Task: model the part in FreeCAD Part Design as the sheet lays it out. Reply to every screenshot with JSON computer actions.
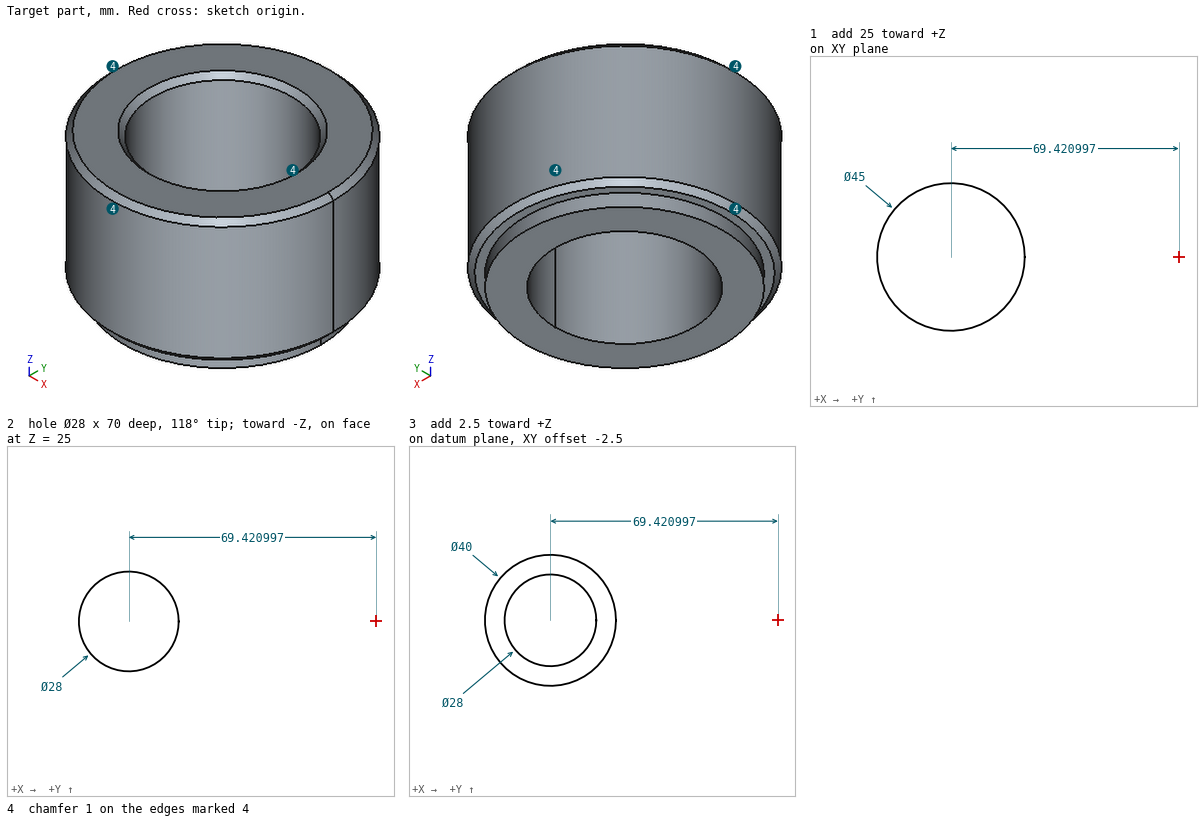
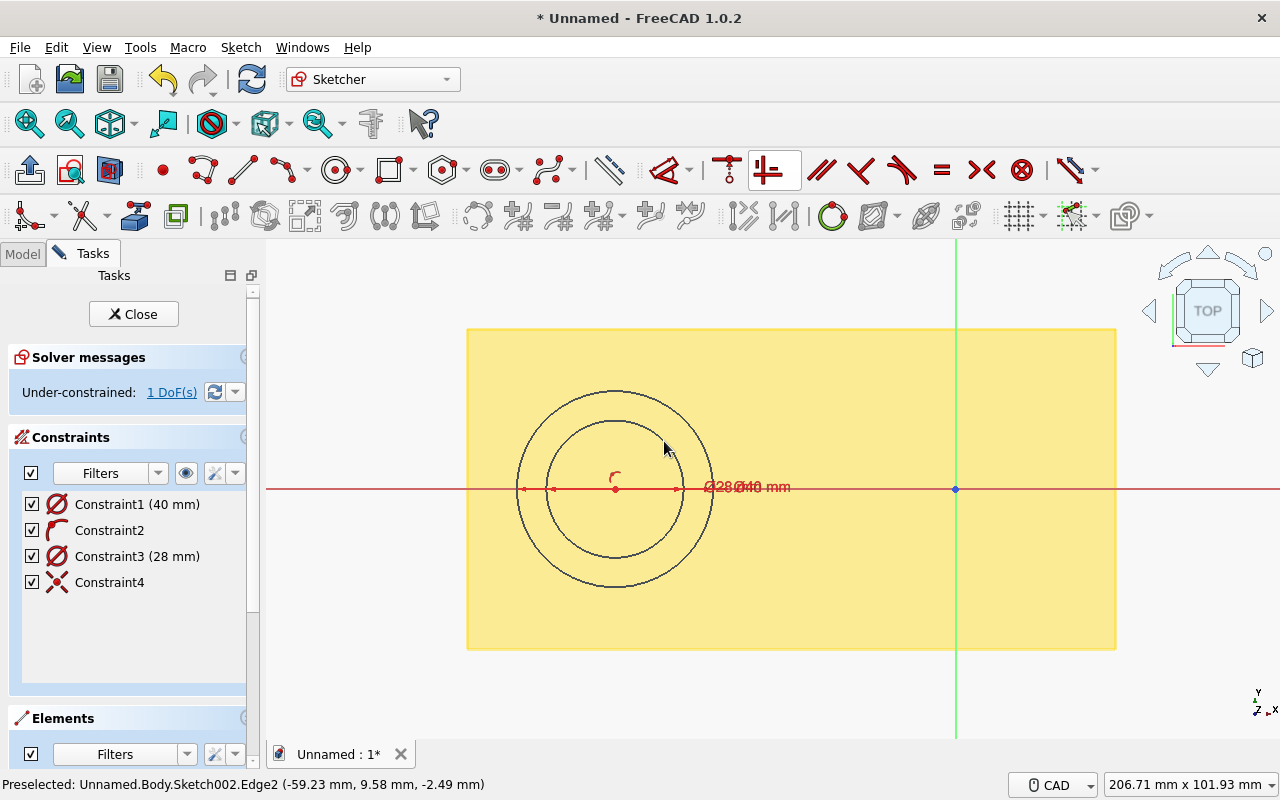
{"action": "key", "text": "d"}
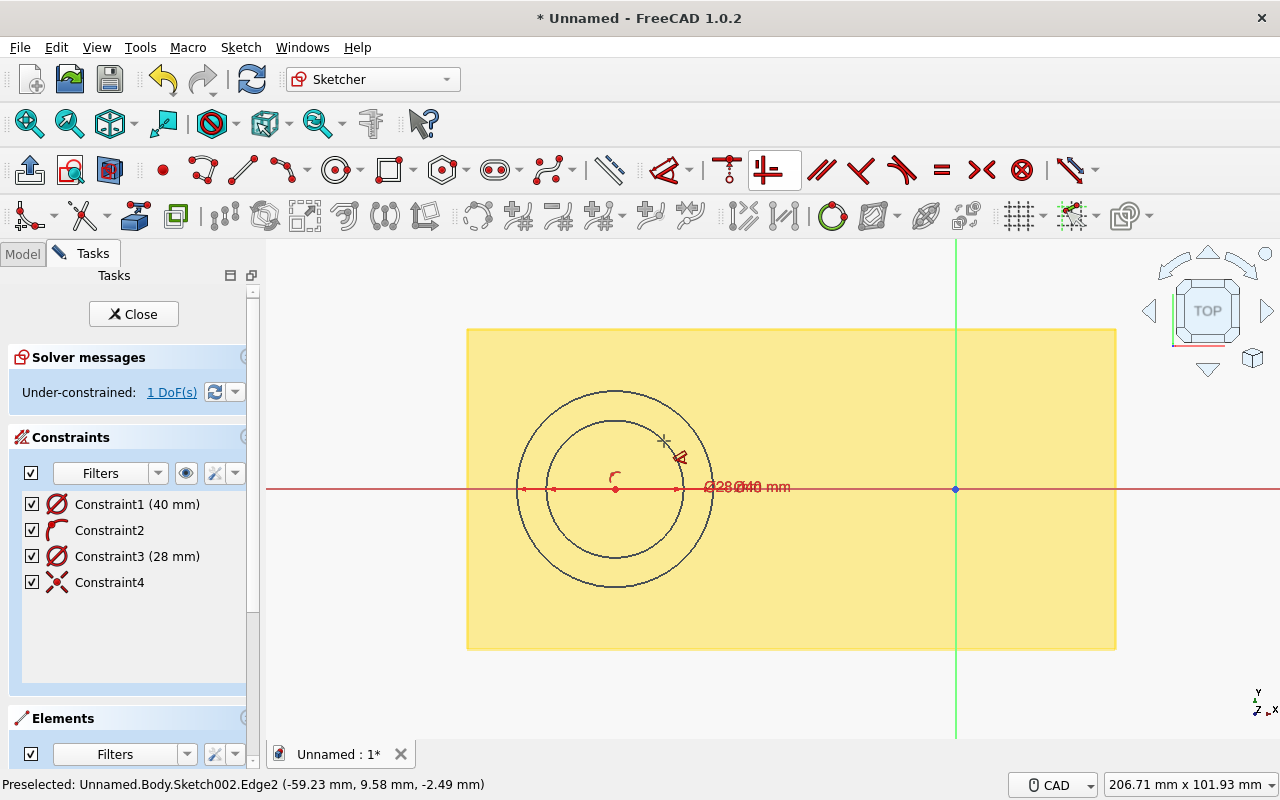
{"action": "left_click", "coordinate": [615, 489]}
{"action": "left_click", "coordinate": [785, 523]}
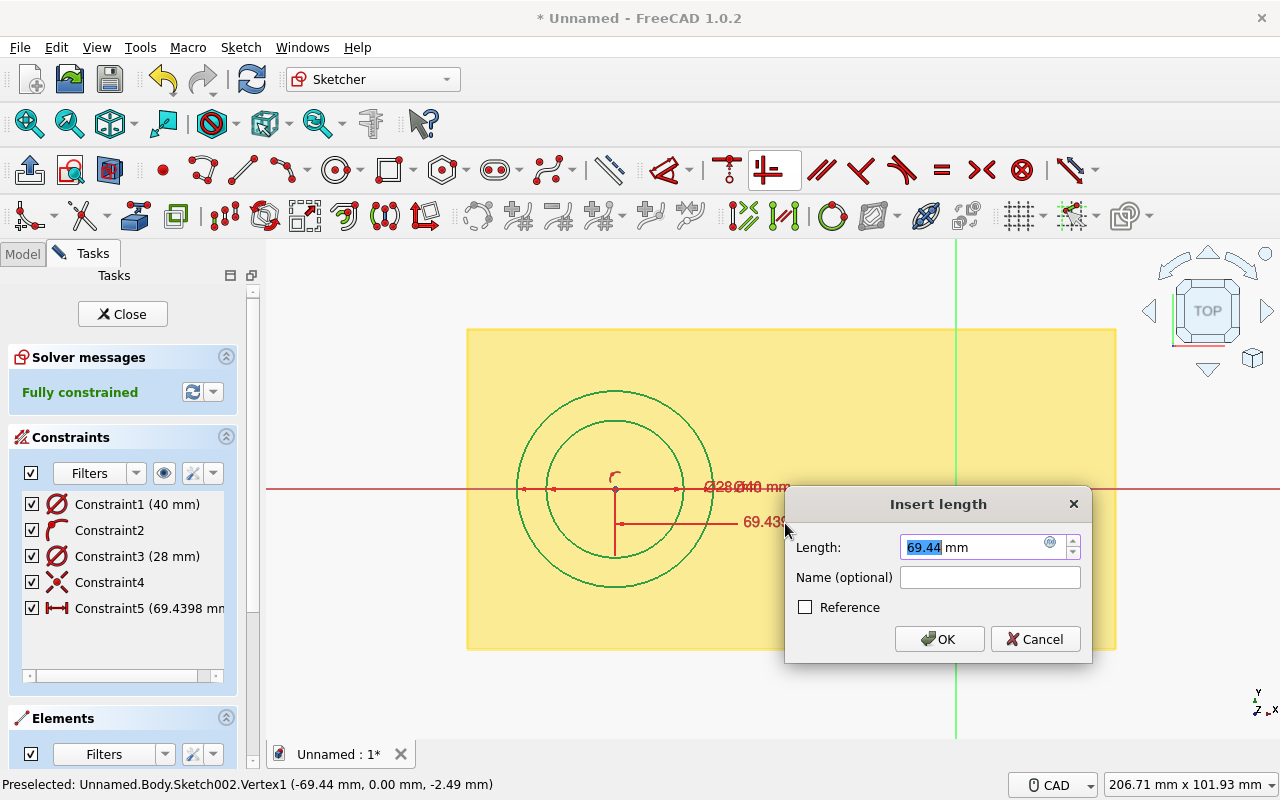
{"action": "type", "text": "69.420997"}
{"action": "key", "text": "Return"}
{"action": "key", "text": "Escape"}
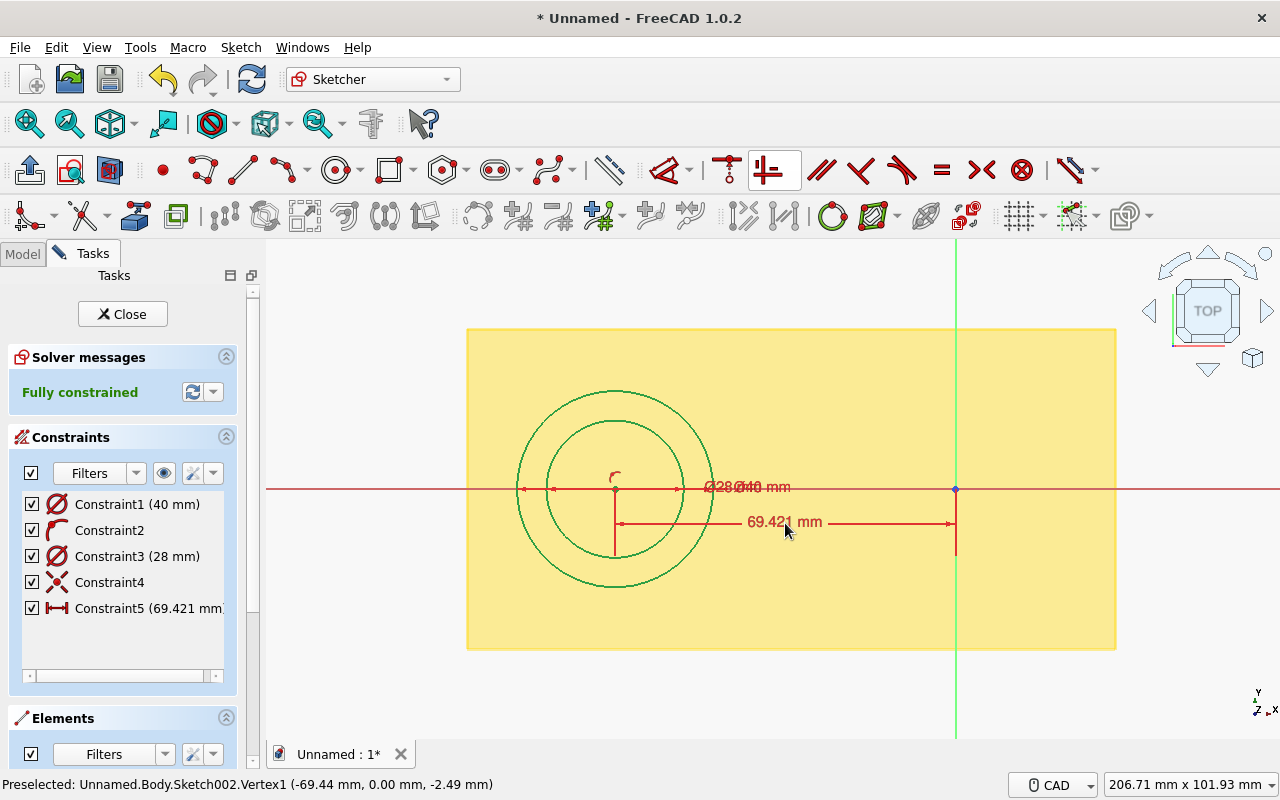
{"action": "left_click", "coordinate": [123, 314]}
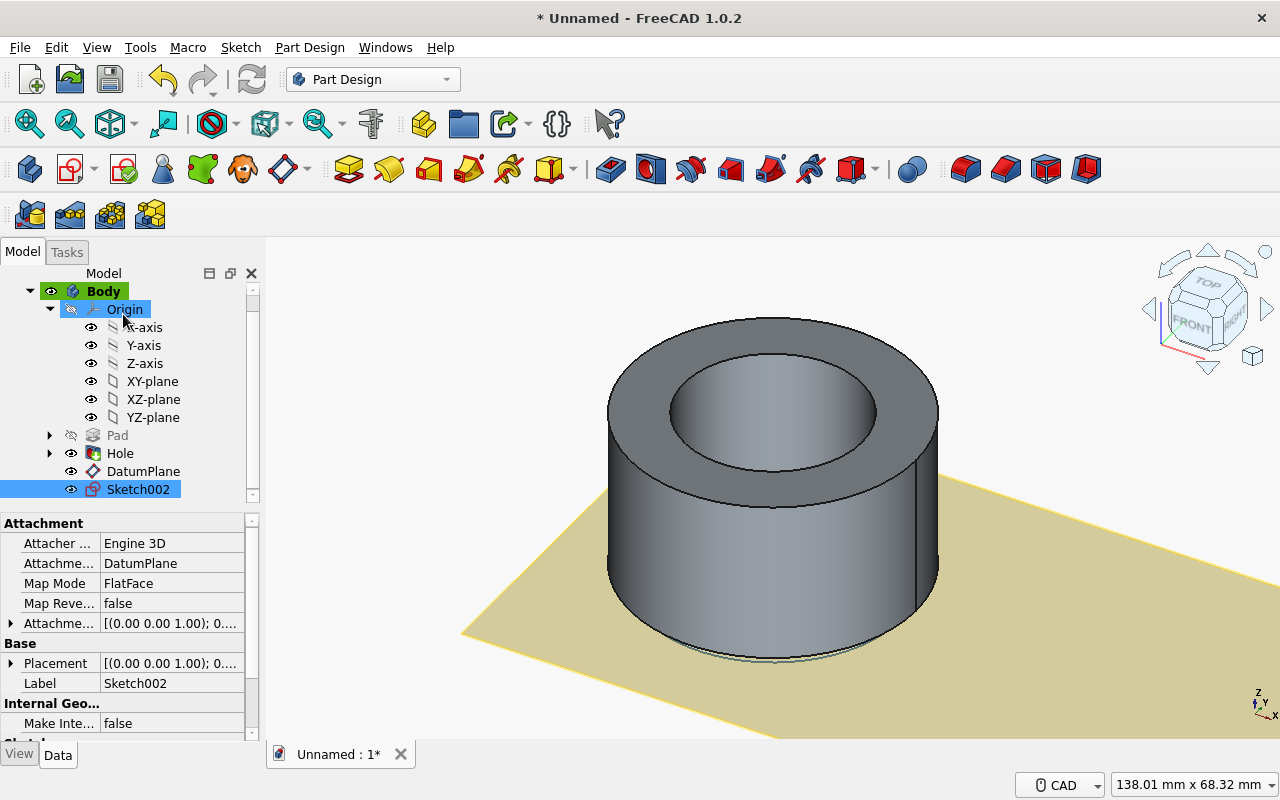
{"action": "left_click", "coordinate": [350, 170]}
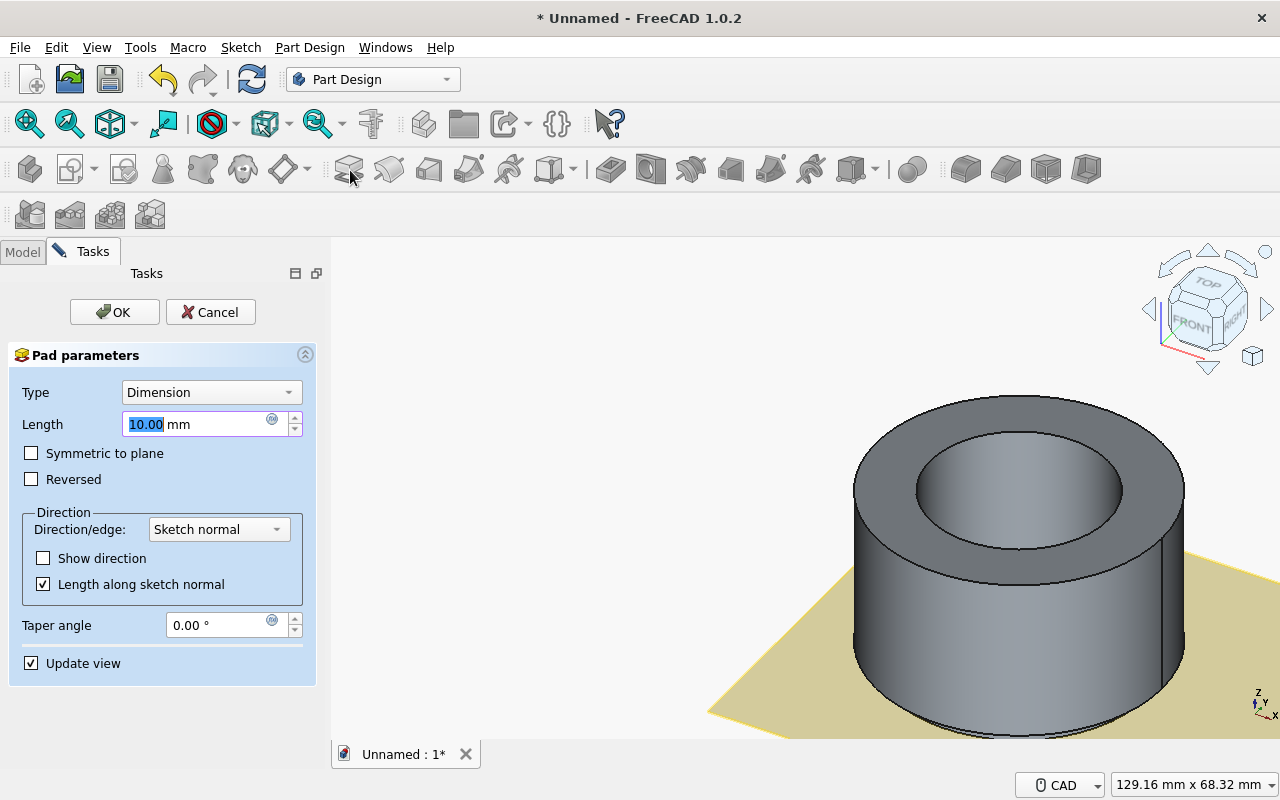
{"action": "type", "text": "2.5"}
{"action": "key", "text": "Tab"}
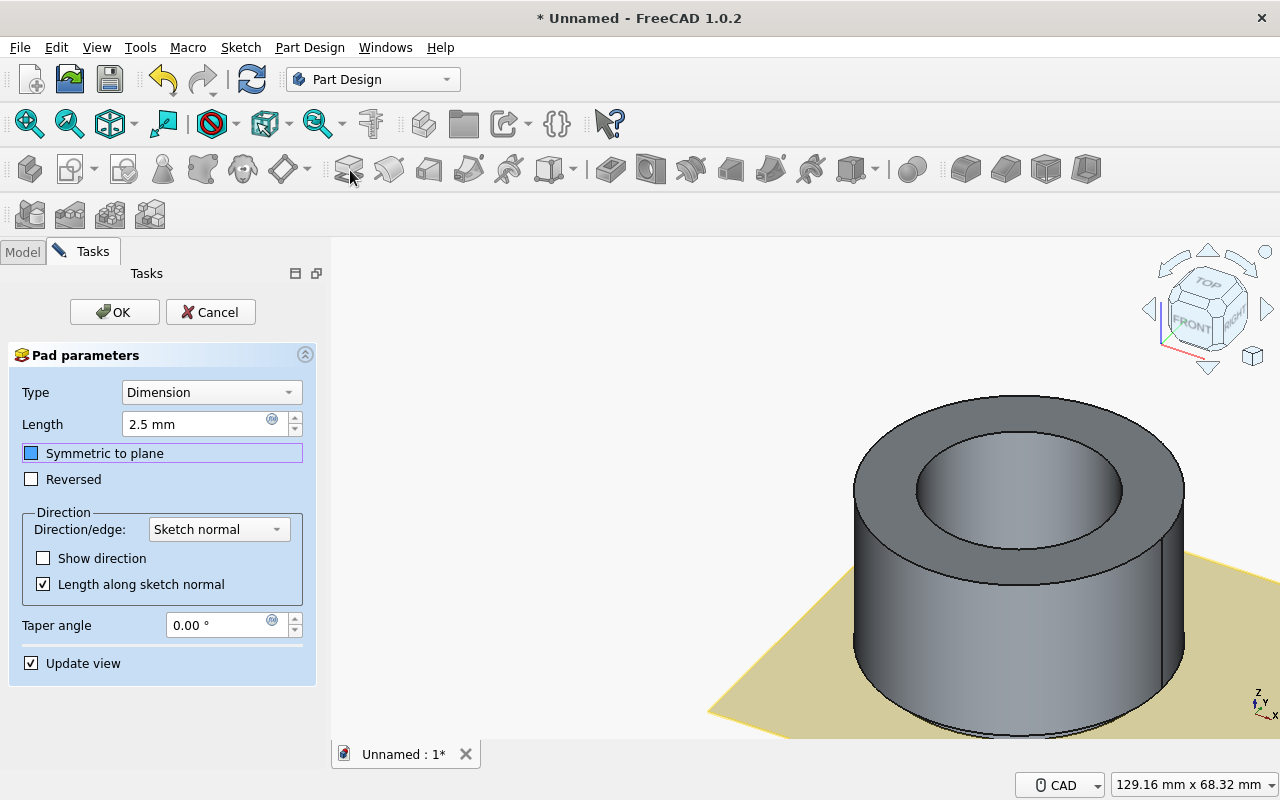
{"action": "left_click", "coordinate": [115, 312]}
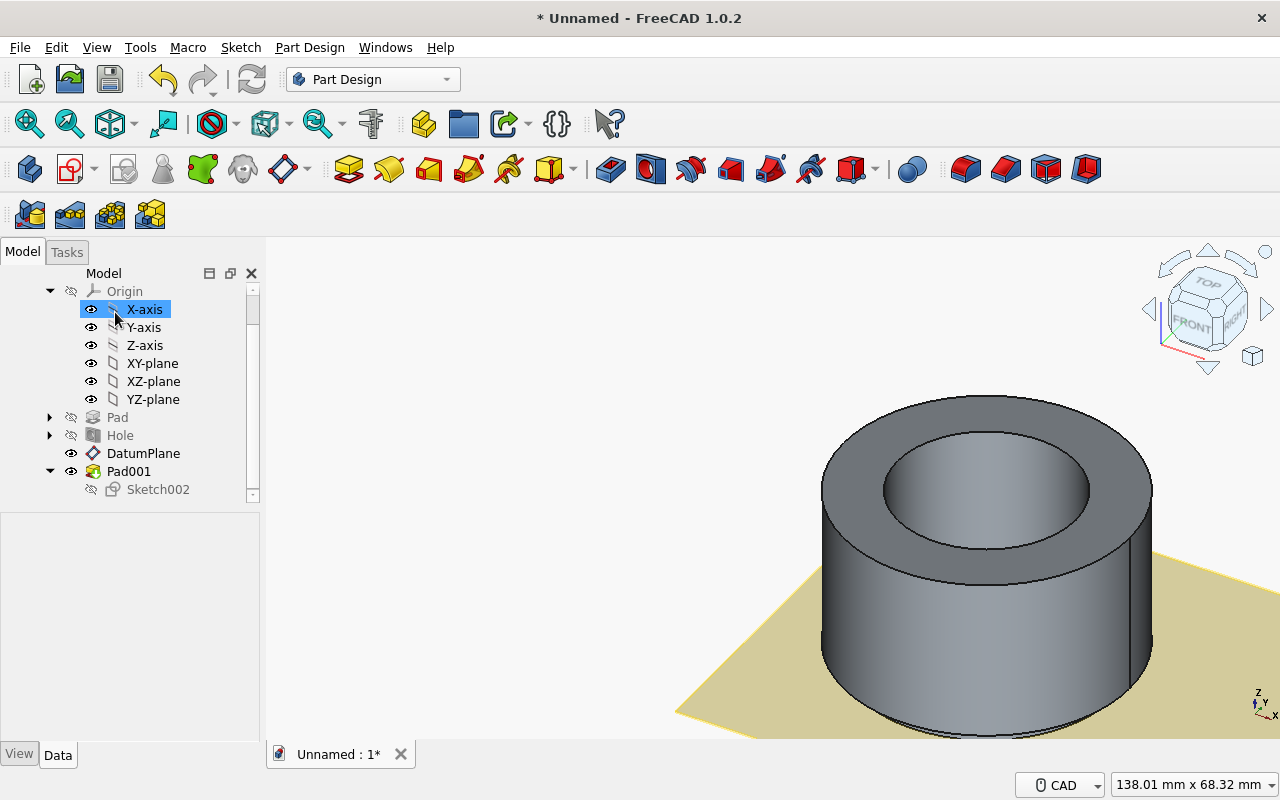
{"action": "left_click", "coordinate": [116, 453]}
{"action": "key", "text": "space"}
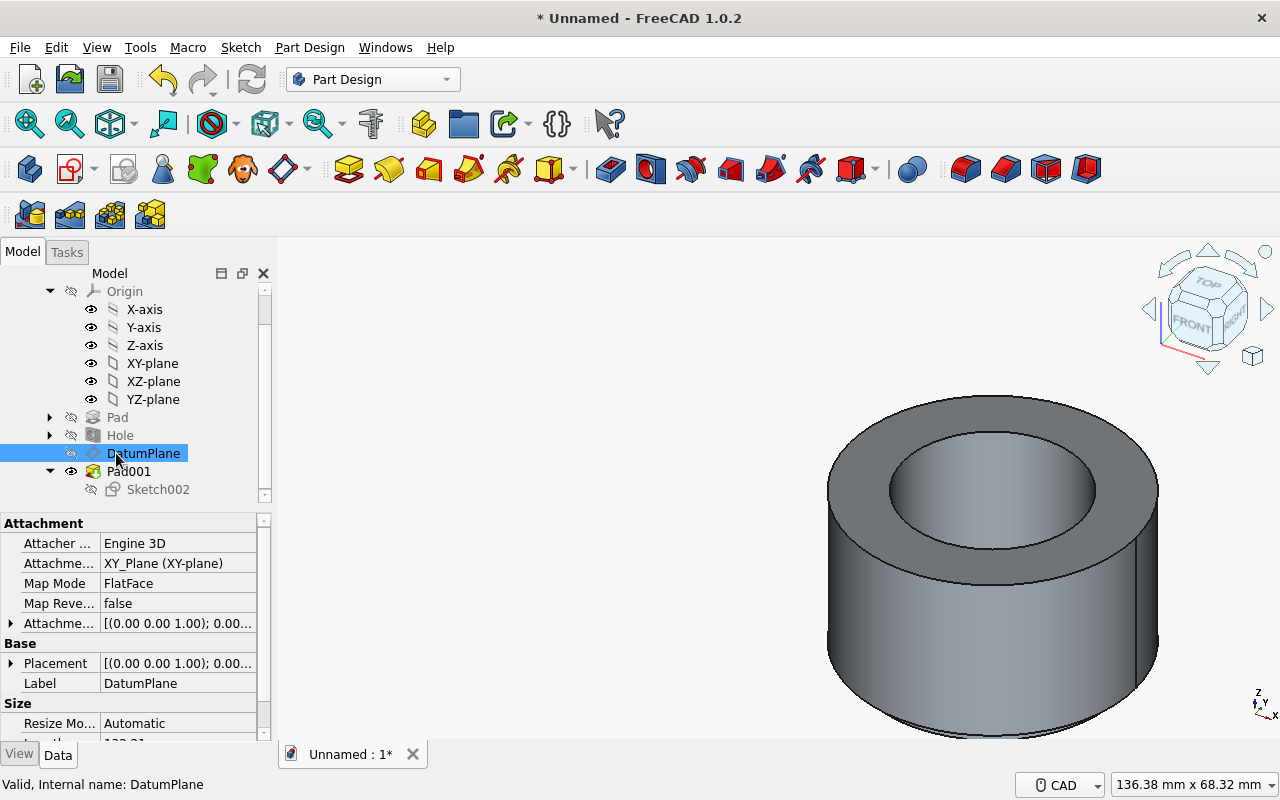
{"action": "key", "text": "v f"}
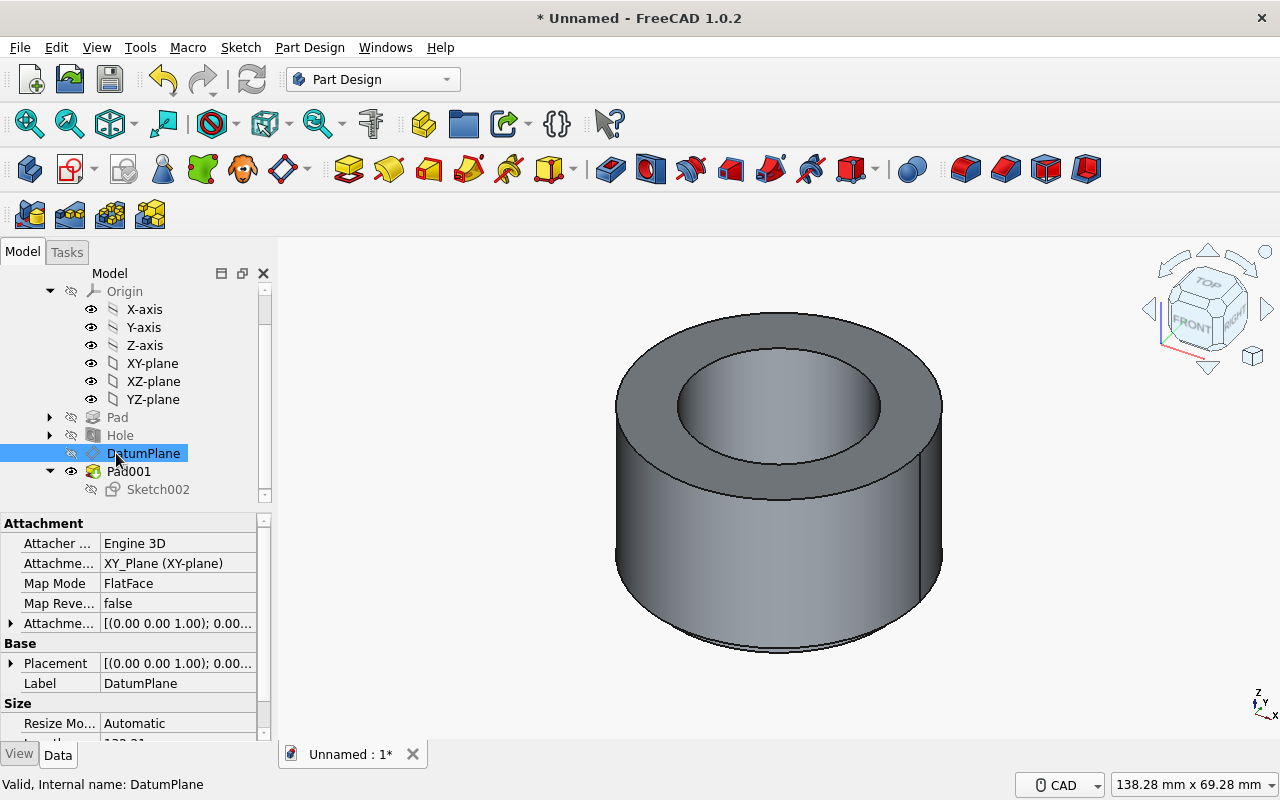
{"action": "left_click", "coordinate": [617, 415]}